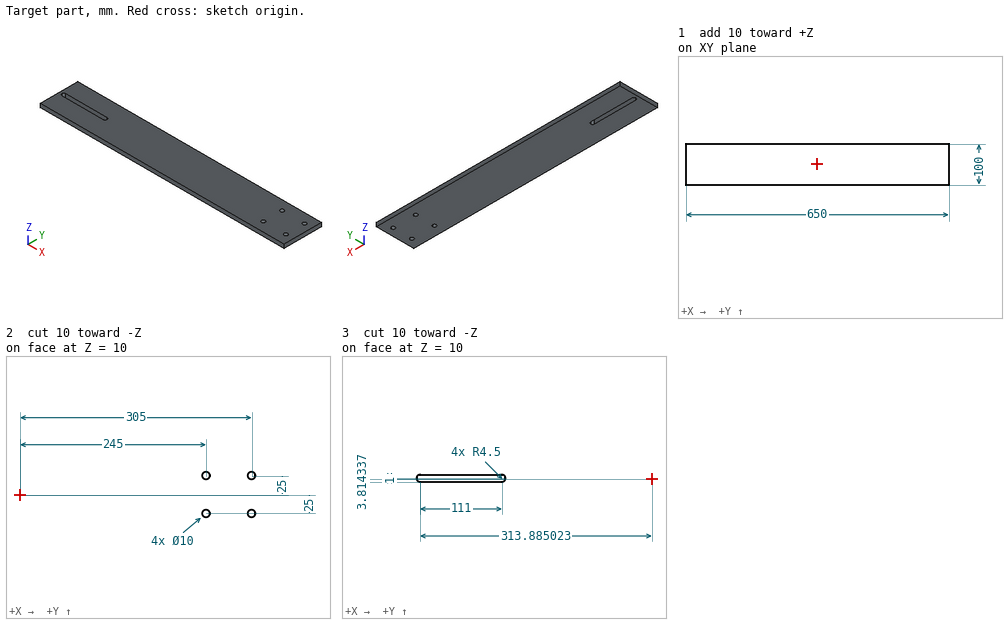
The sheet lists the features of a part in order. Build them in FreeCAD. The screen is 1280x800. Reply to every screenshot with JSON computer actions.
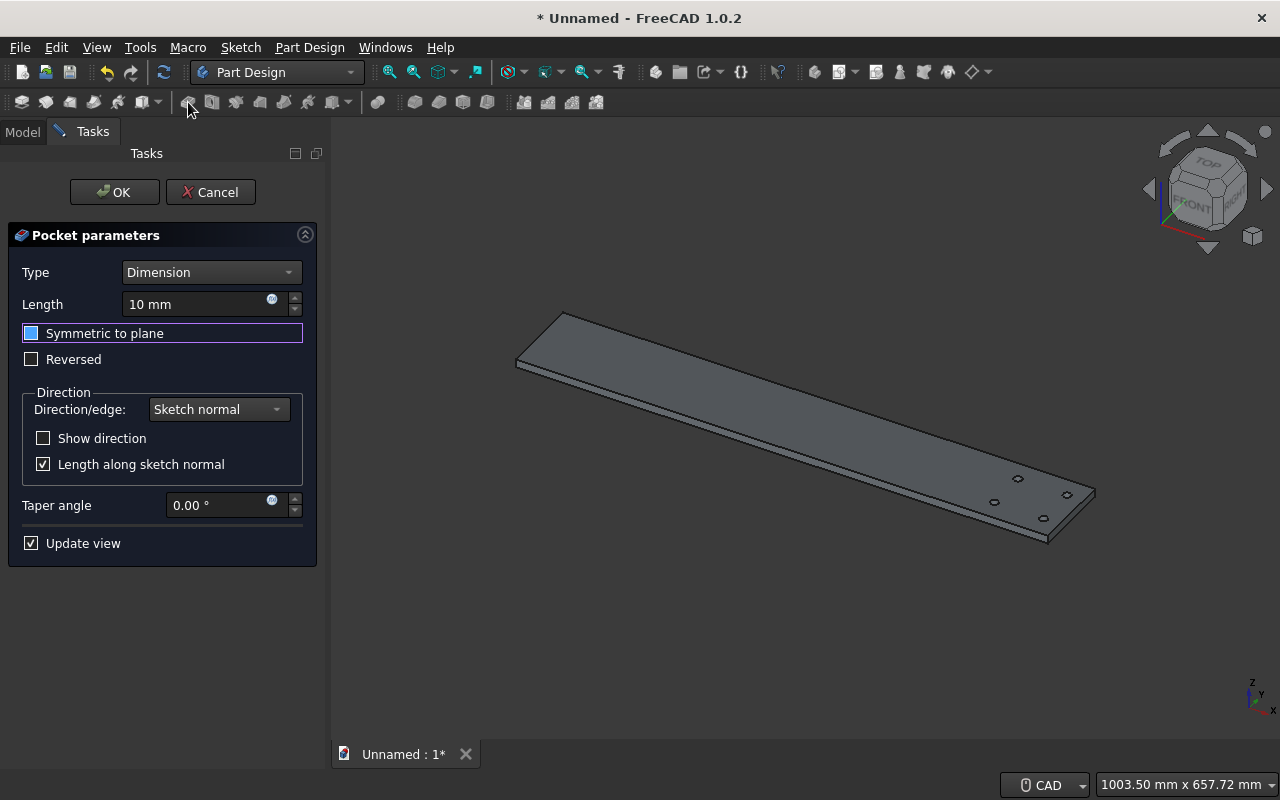
{"action": "left_click", "coordinate": [115, 192]}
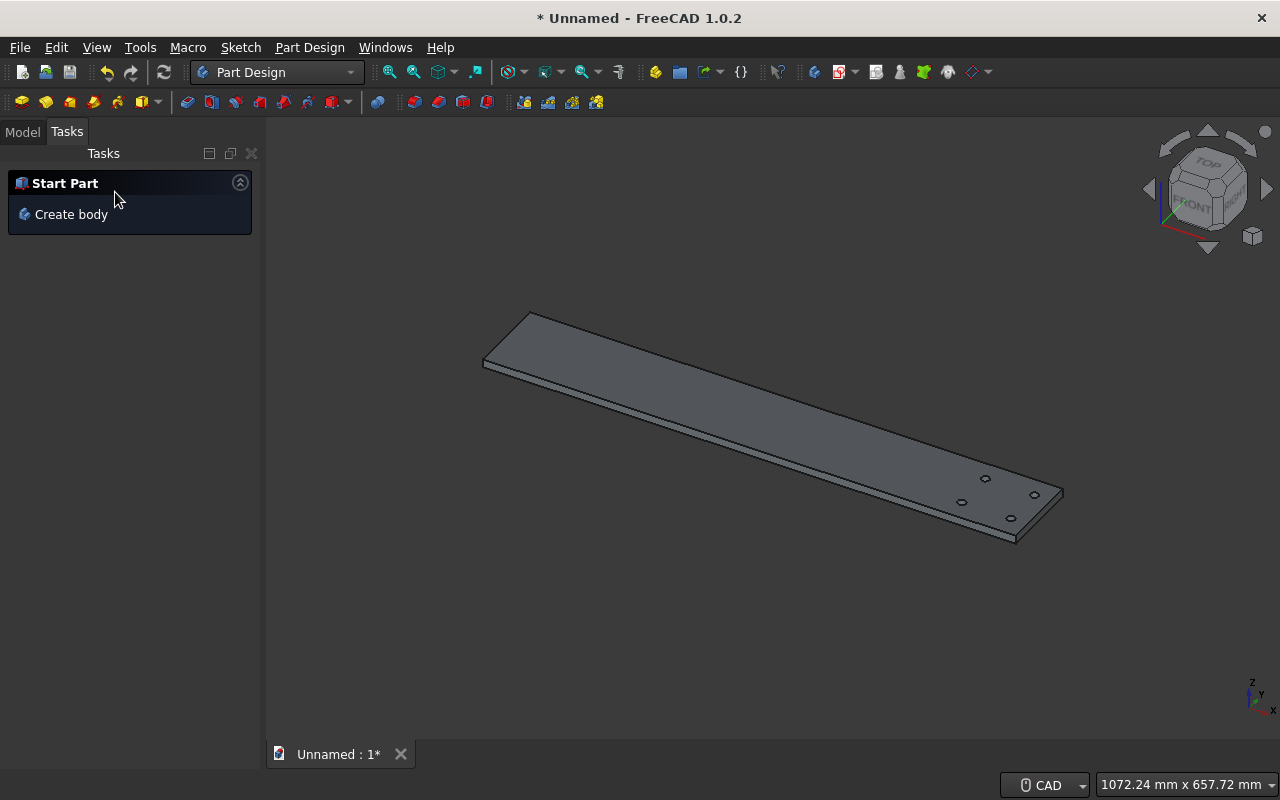
{"action": "left_click", "coordinate": [925, 473]}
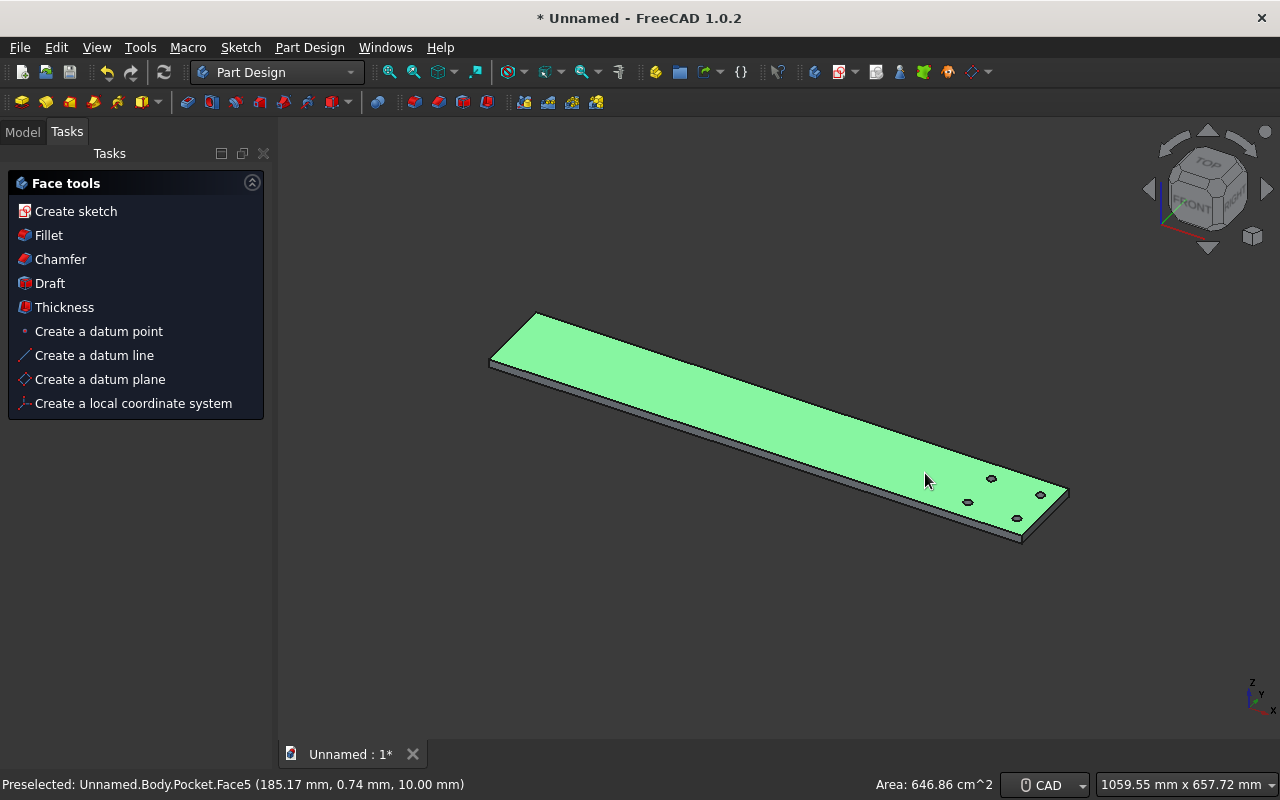
{"action": "left_click", "coordinate": [840, 72]}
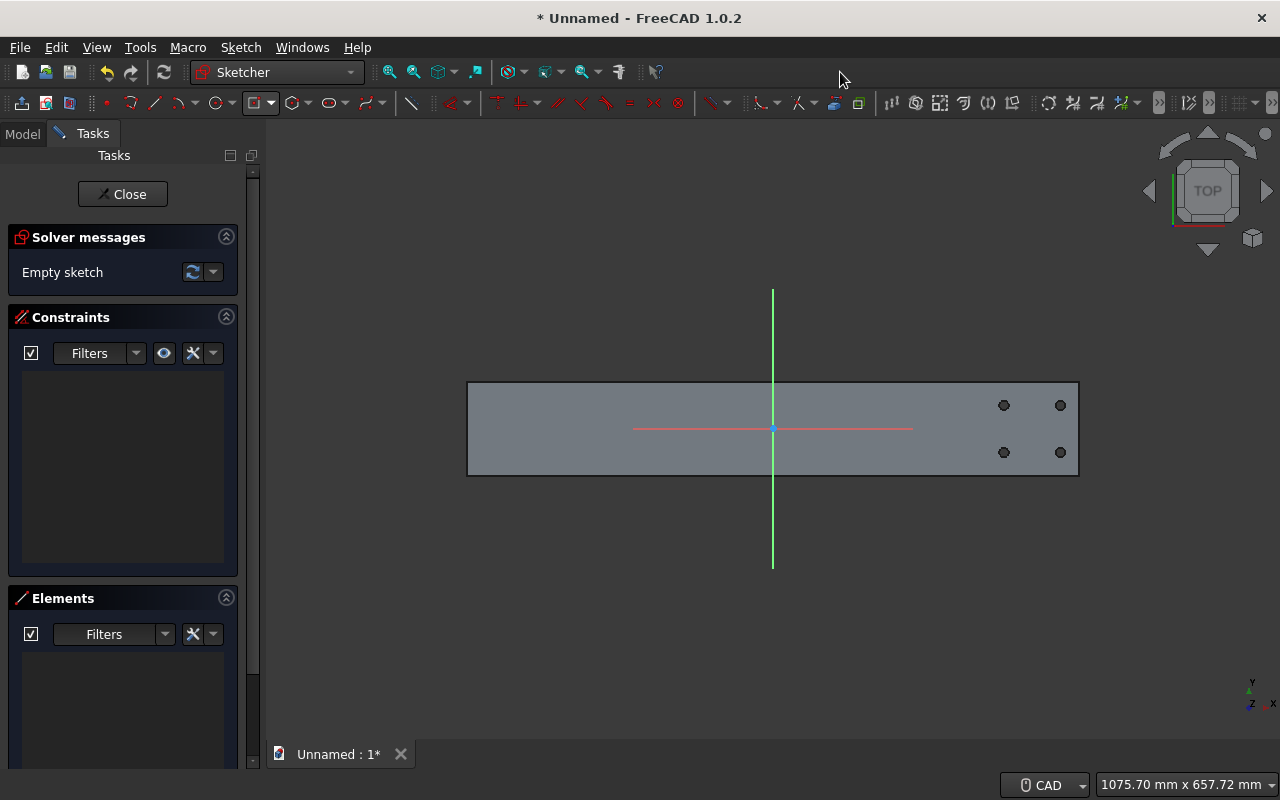
{"action": "scroll", "coordinate": [485, 428], "scroll_direction": "up", "scroll_amount": 8}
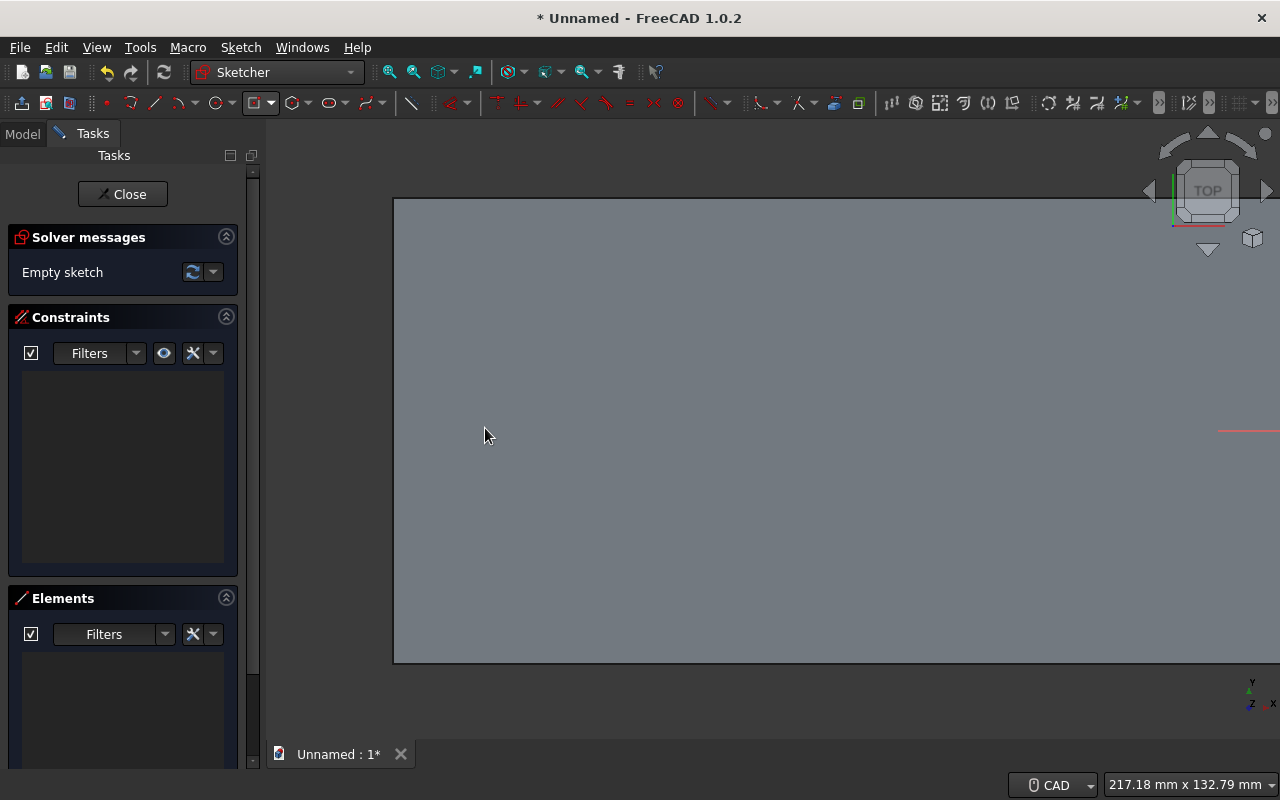
{"action": "key", "text": "g l"}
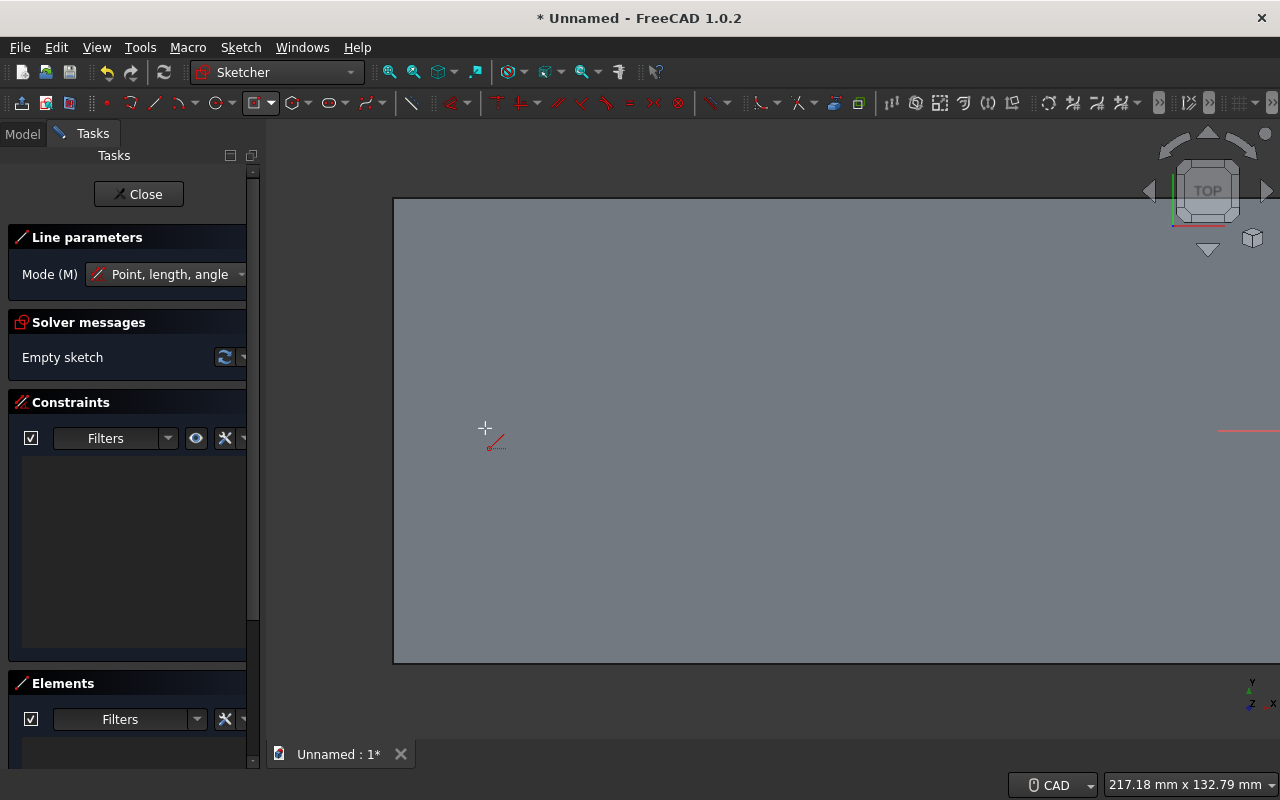
{"action": "left_click", "coordinate": [445, 449]}
{"action": "left_click", "coordinate": [963, 449]}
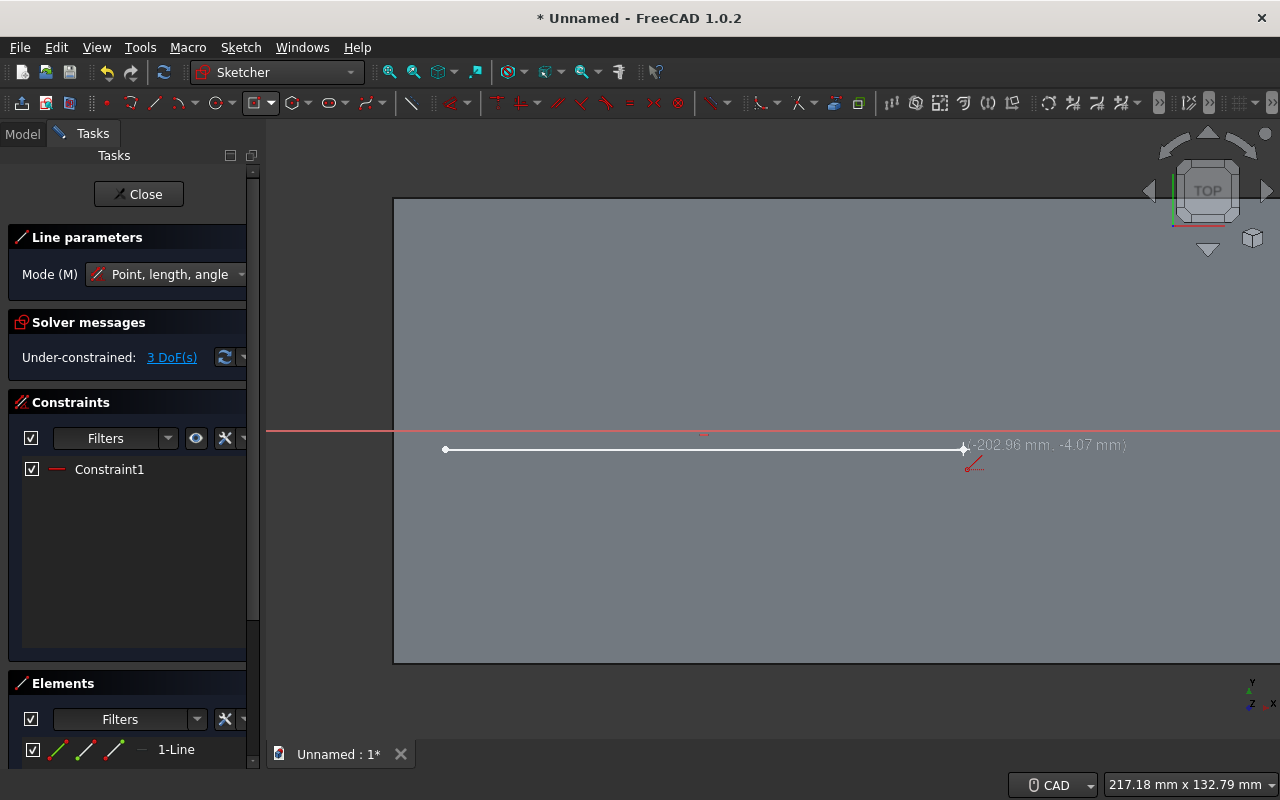
{"action": "scroll", "coordinate": [984, 428], "scroll_direction": "up", "scroll_amount": 9}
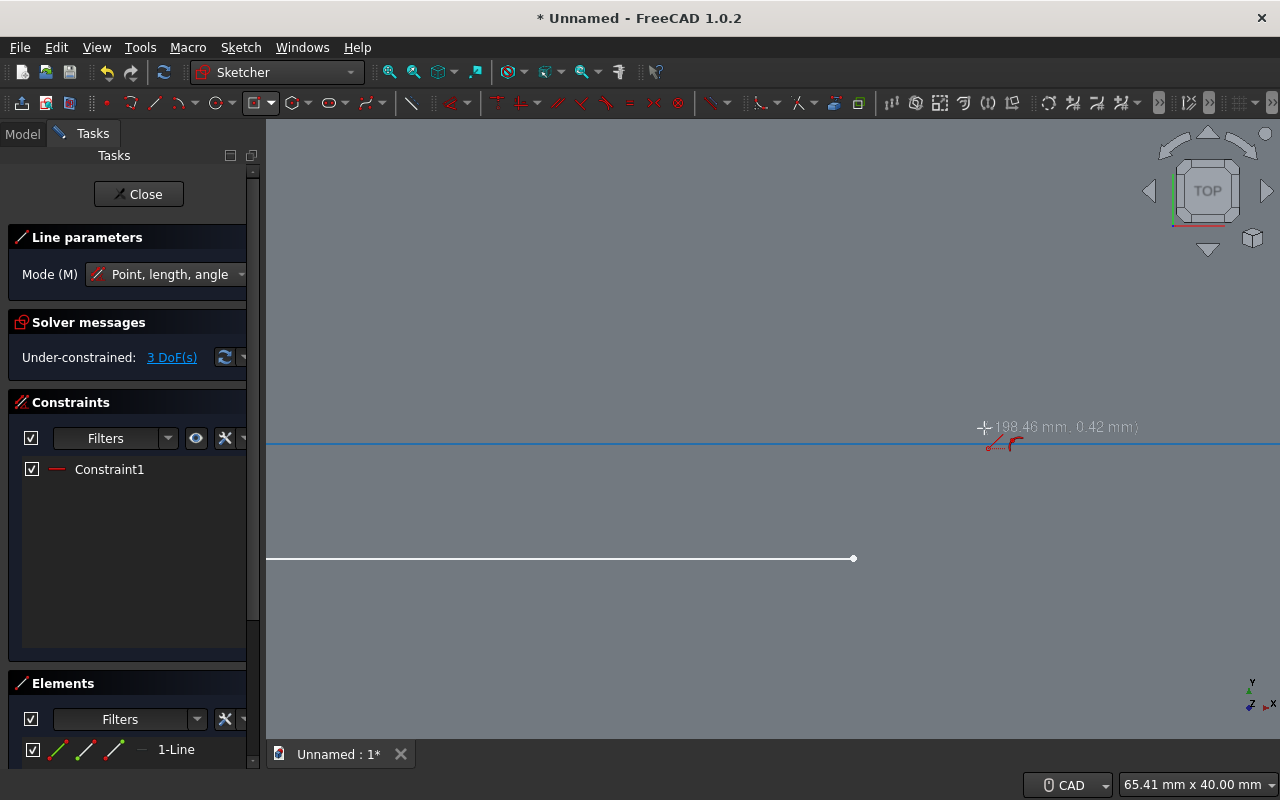
{"action": "left_click", "coordinate": [983, 424]}
{"action": "left_click", "coordinate": [983, 396]}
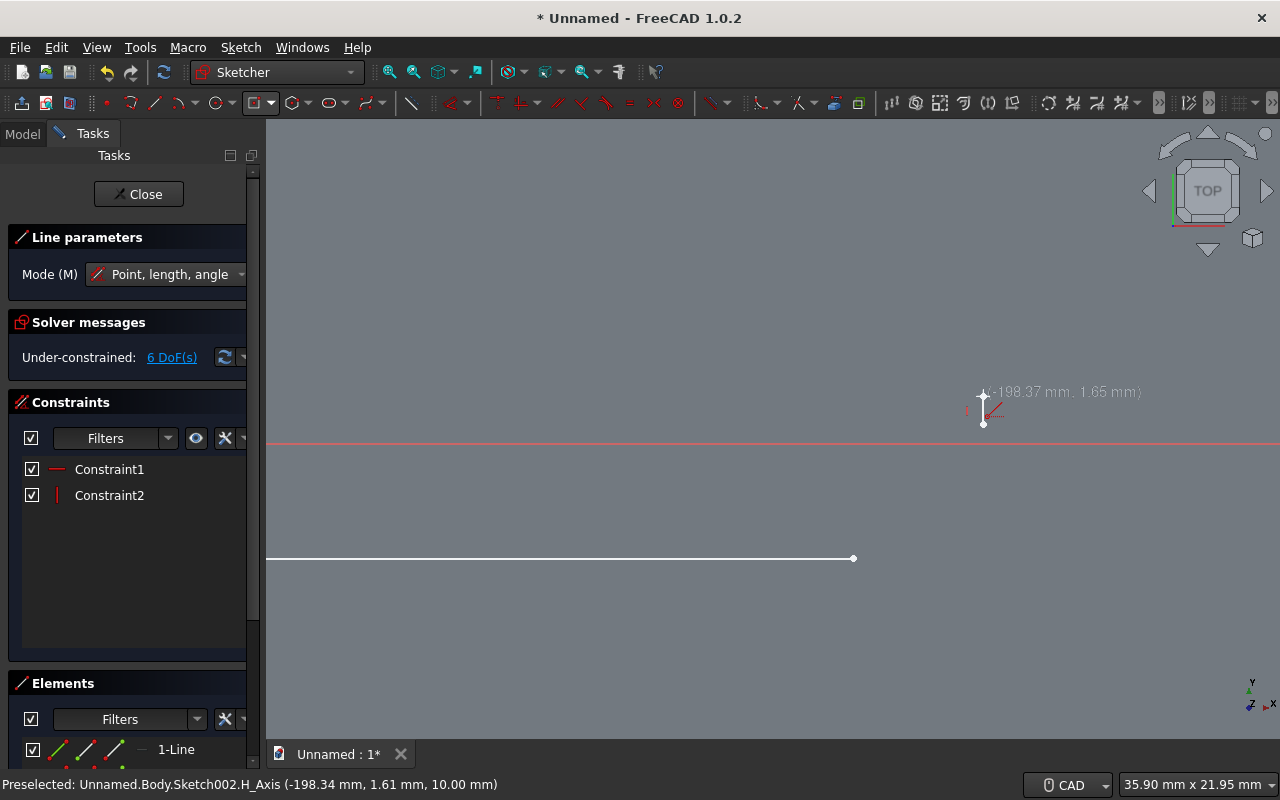
{"action": "scroll", "coordinate": [985, 433], "scroll_direction": "down", "scroll_amount": 9}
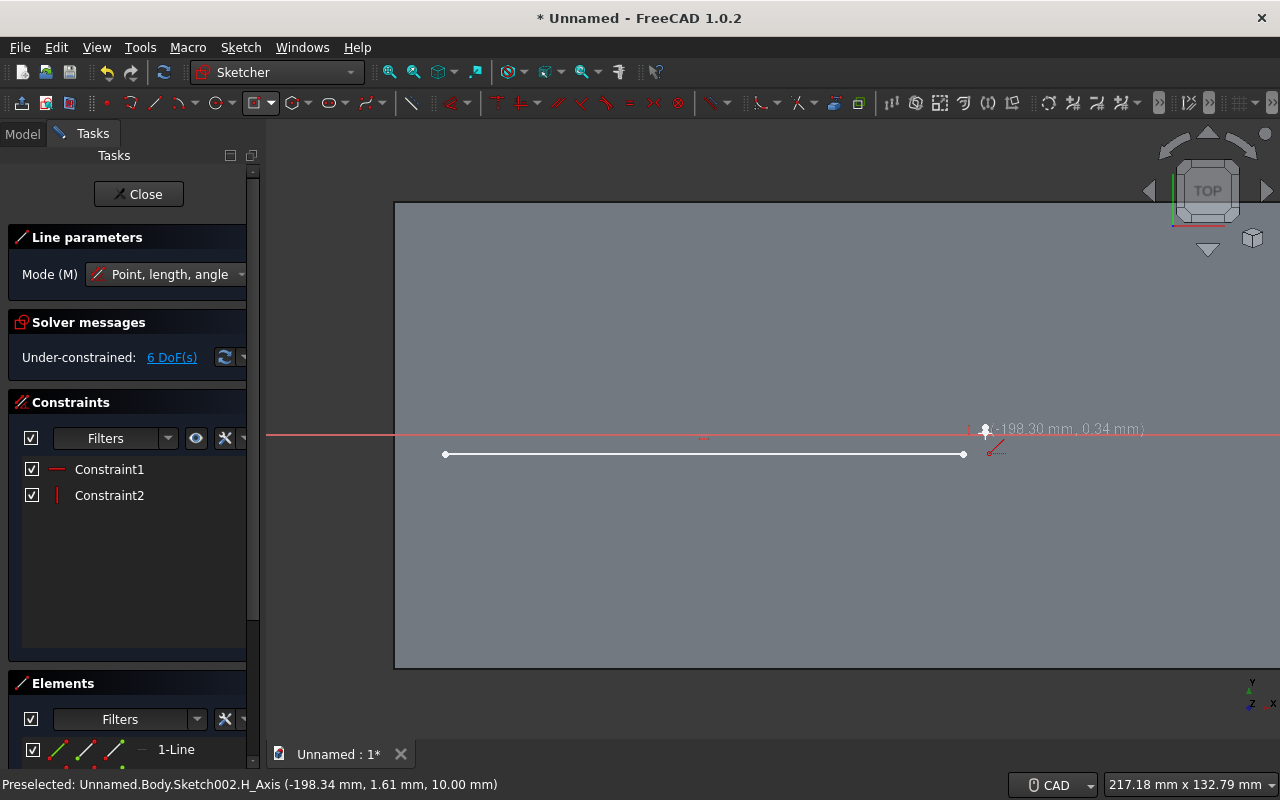
{"action": "left_click", "coordinate": [964, 406]}
{"action": "left_click", "coordinate": [446, 406]}